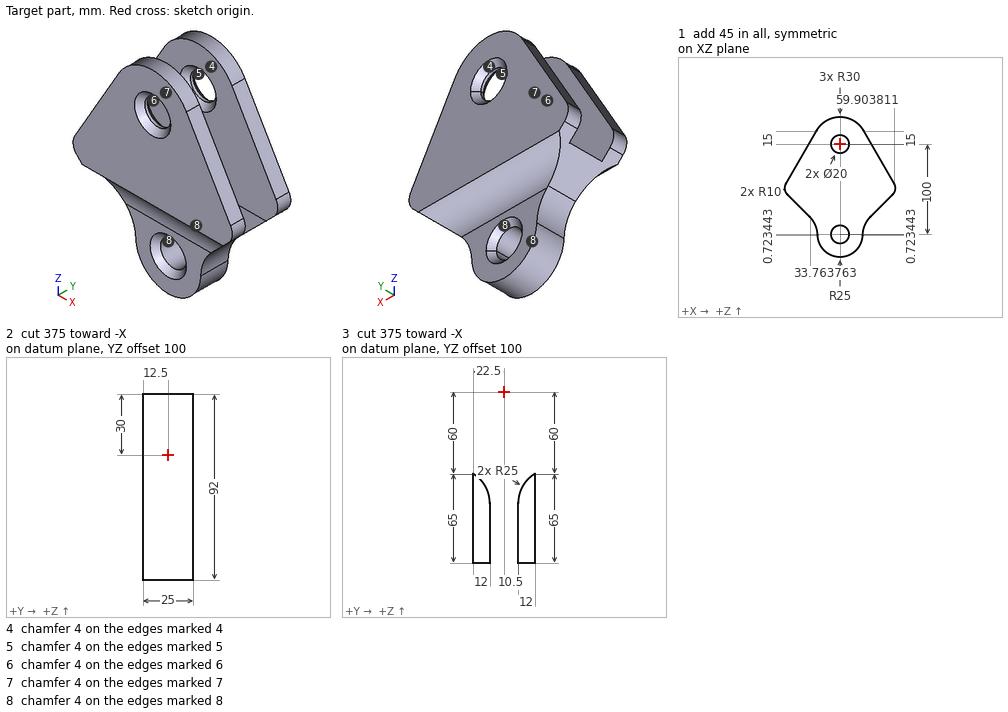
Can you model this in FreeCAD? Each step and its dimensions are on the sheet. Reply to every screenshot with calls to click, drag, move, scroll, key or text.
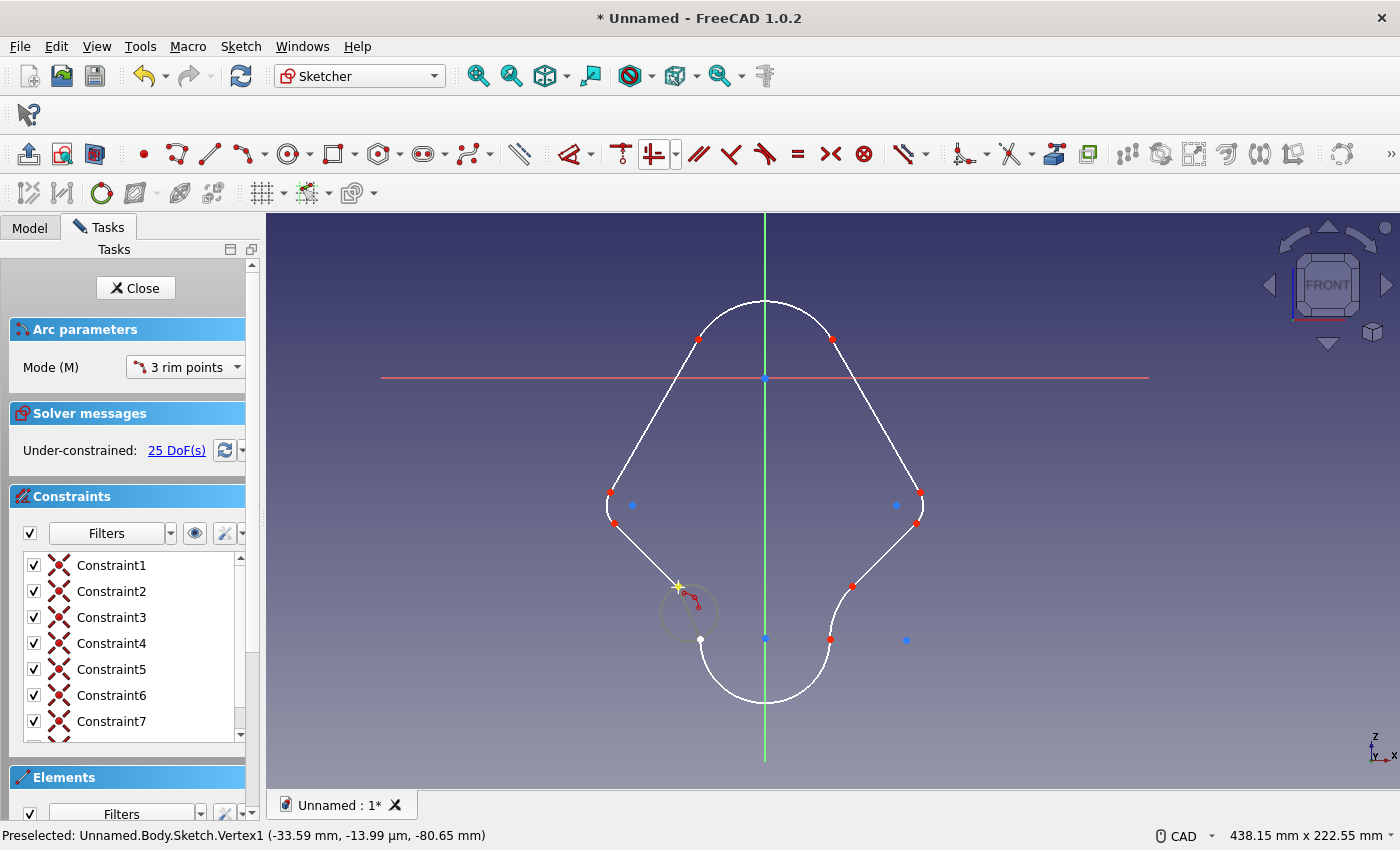
scroll(694, 610, up, 6)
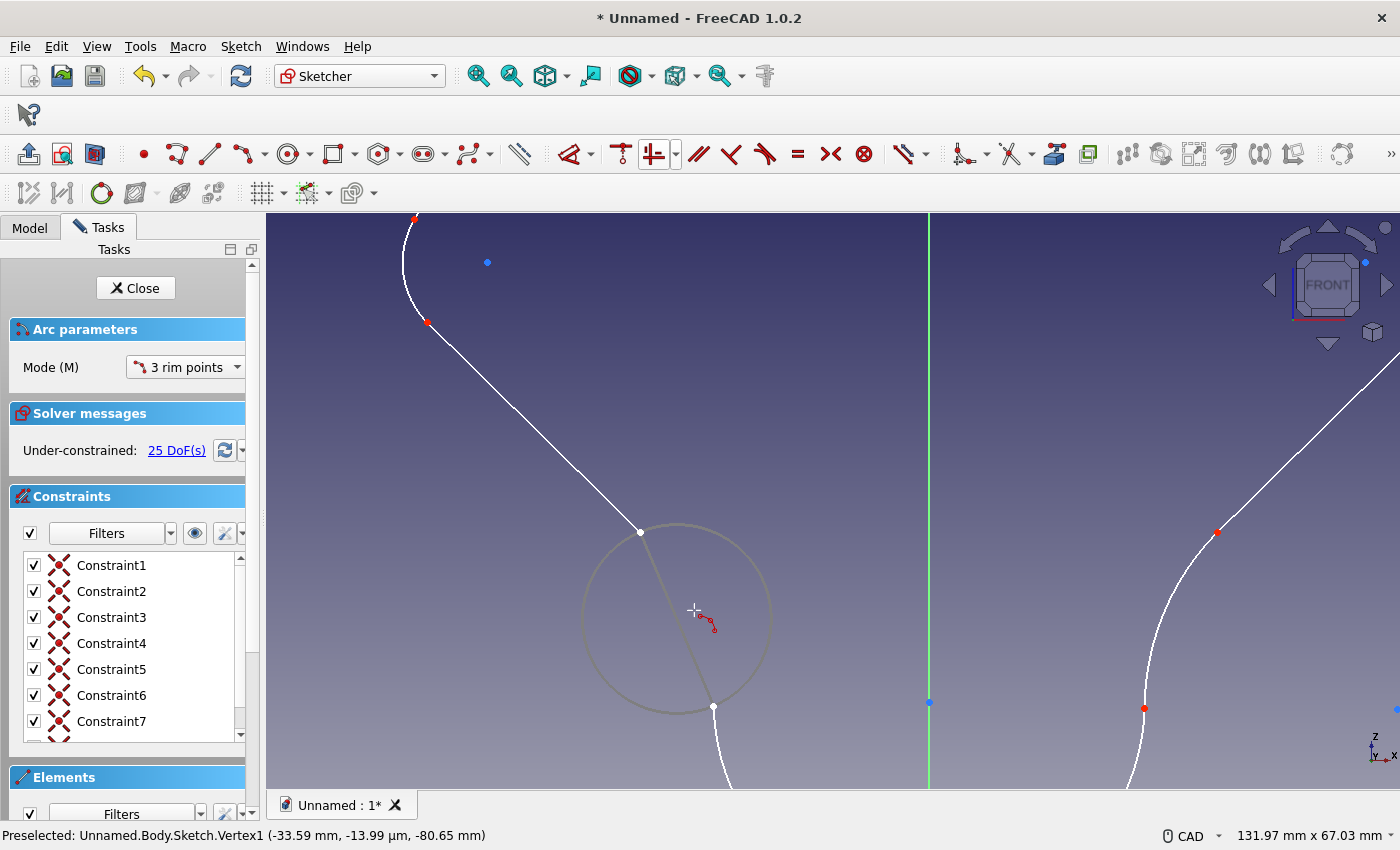
click(693, 610)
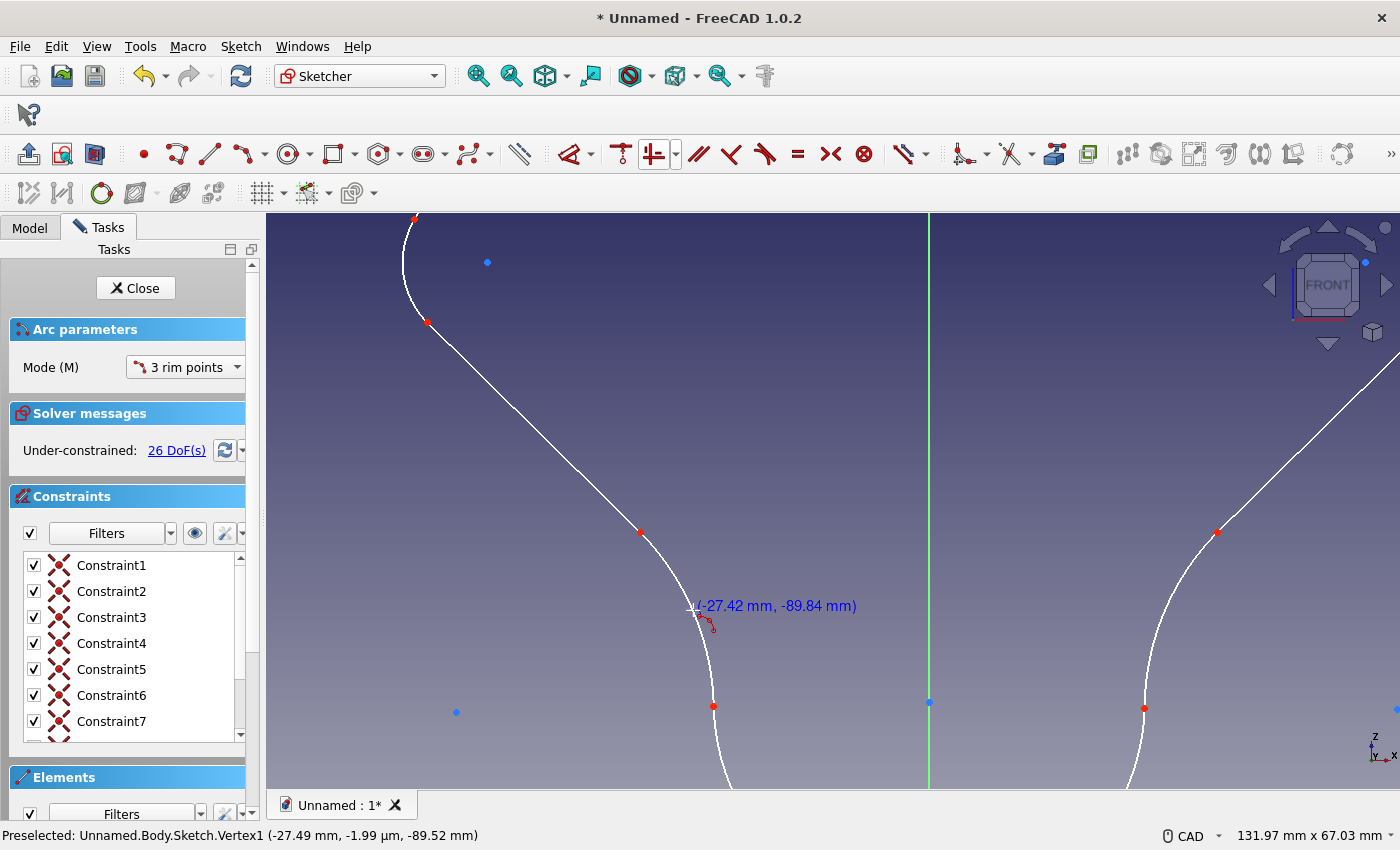
click(288, 154)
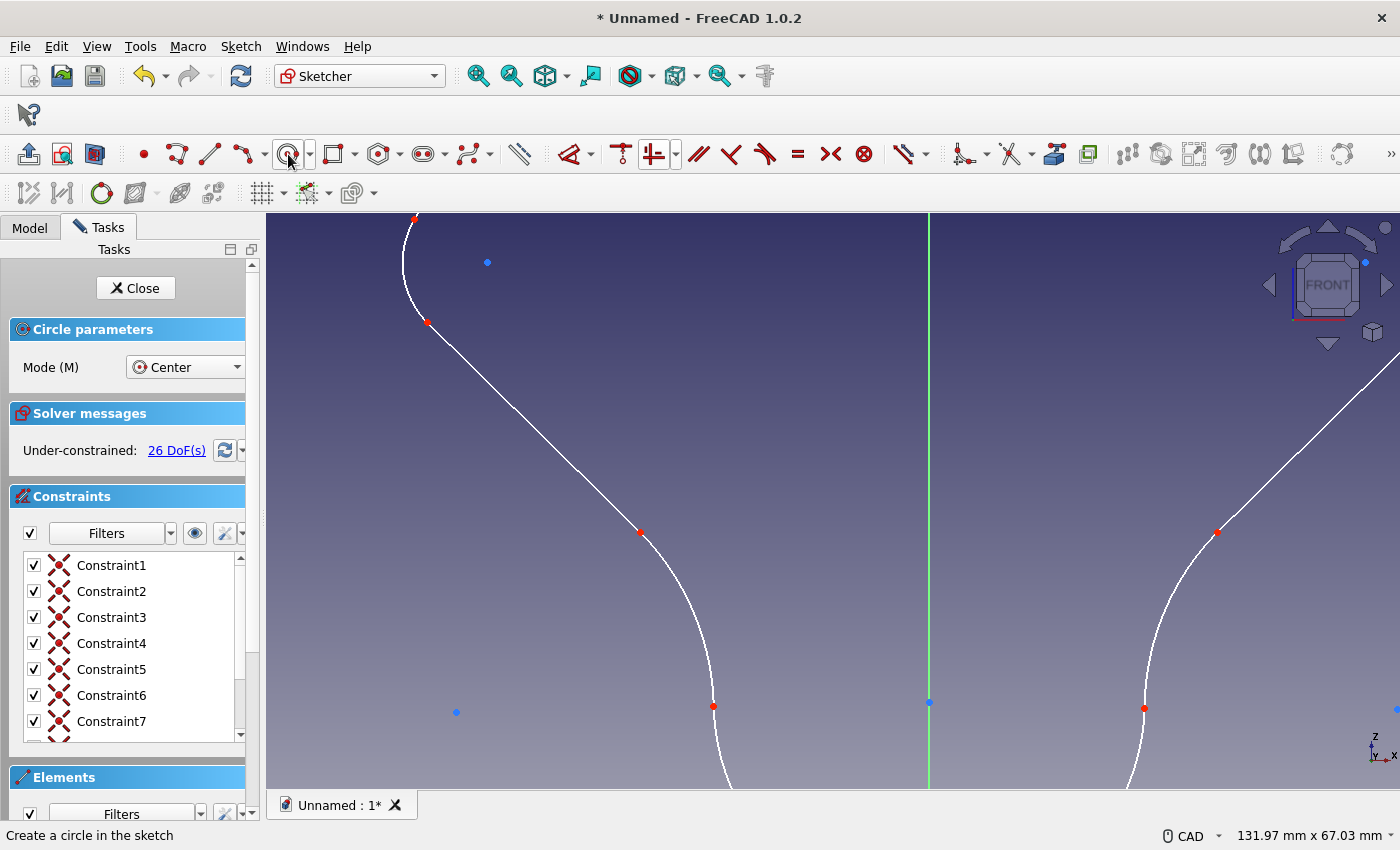
scroll(694, 610, down, 6)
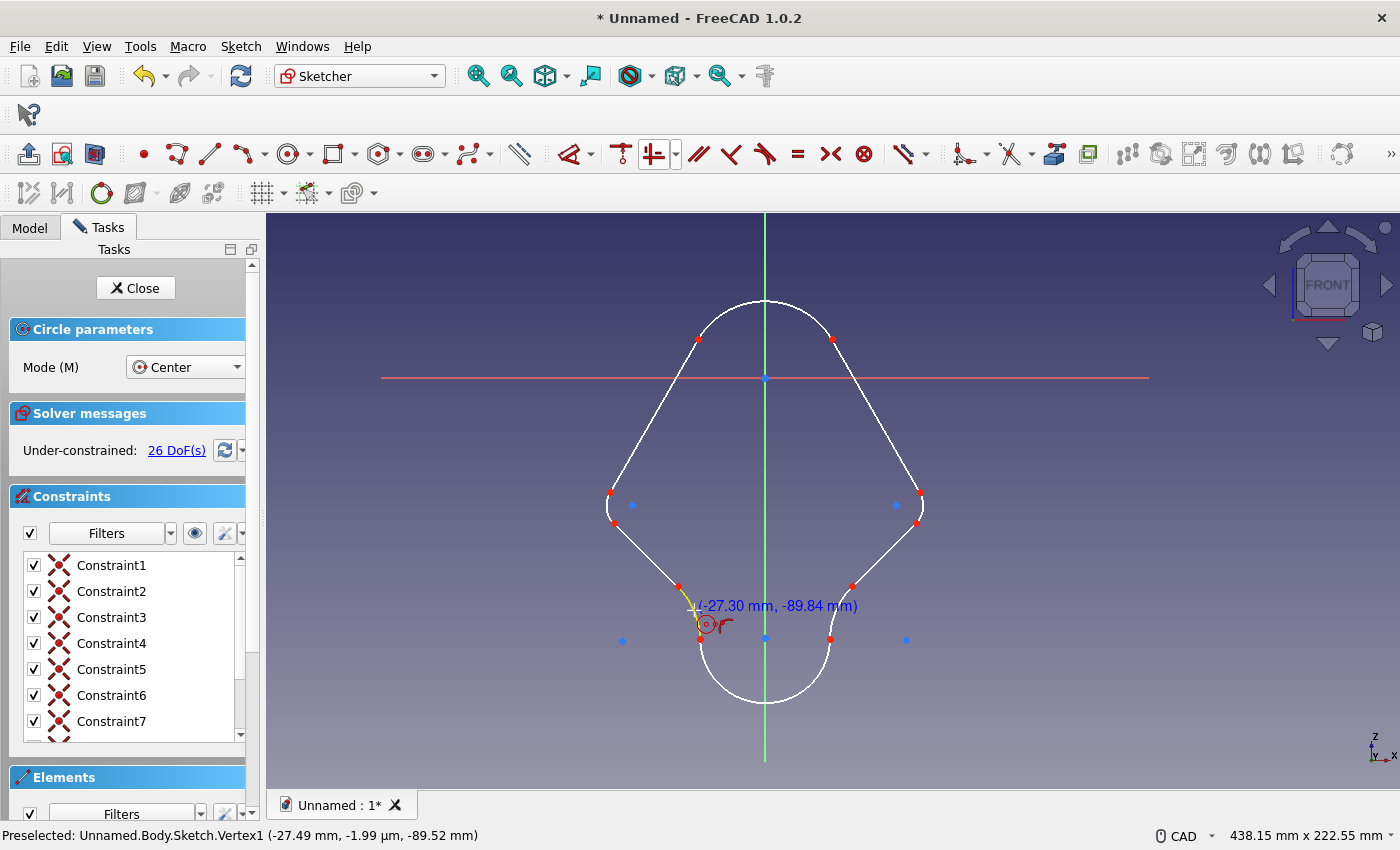
click(765, 378)
move(783, 360)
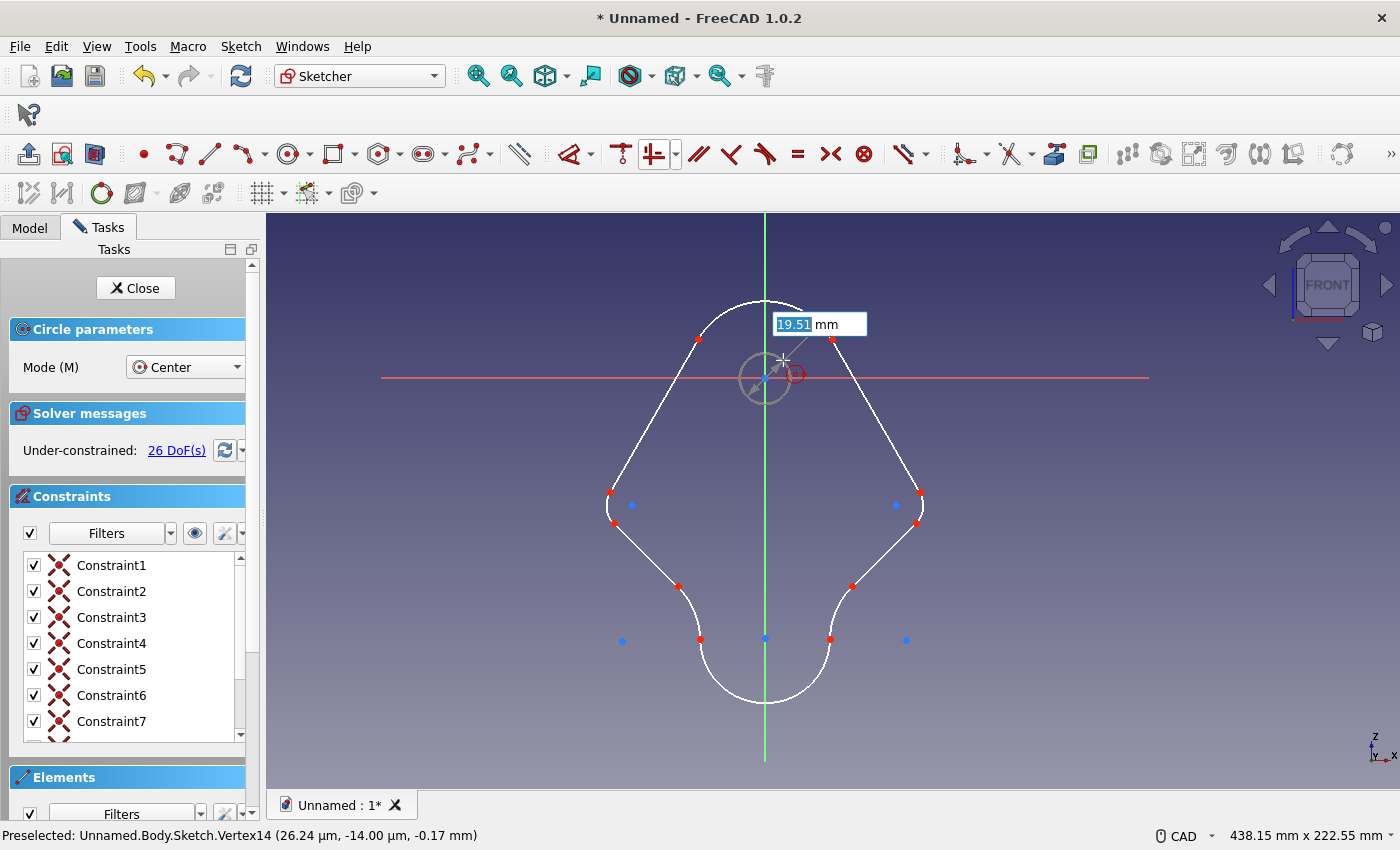
text(20)
key(Return)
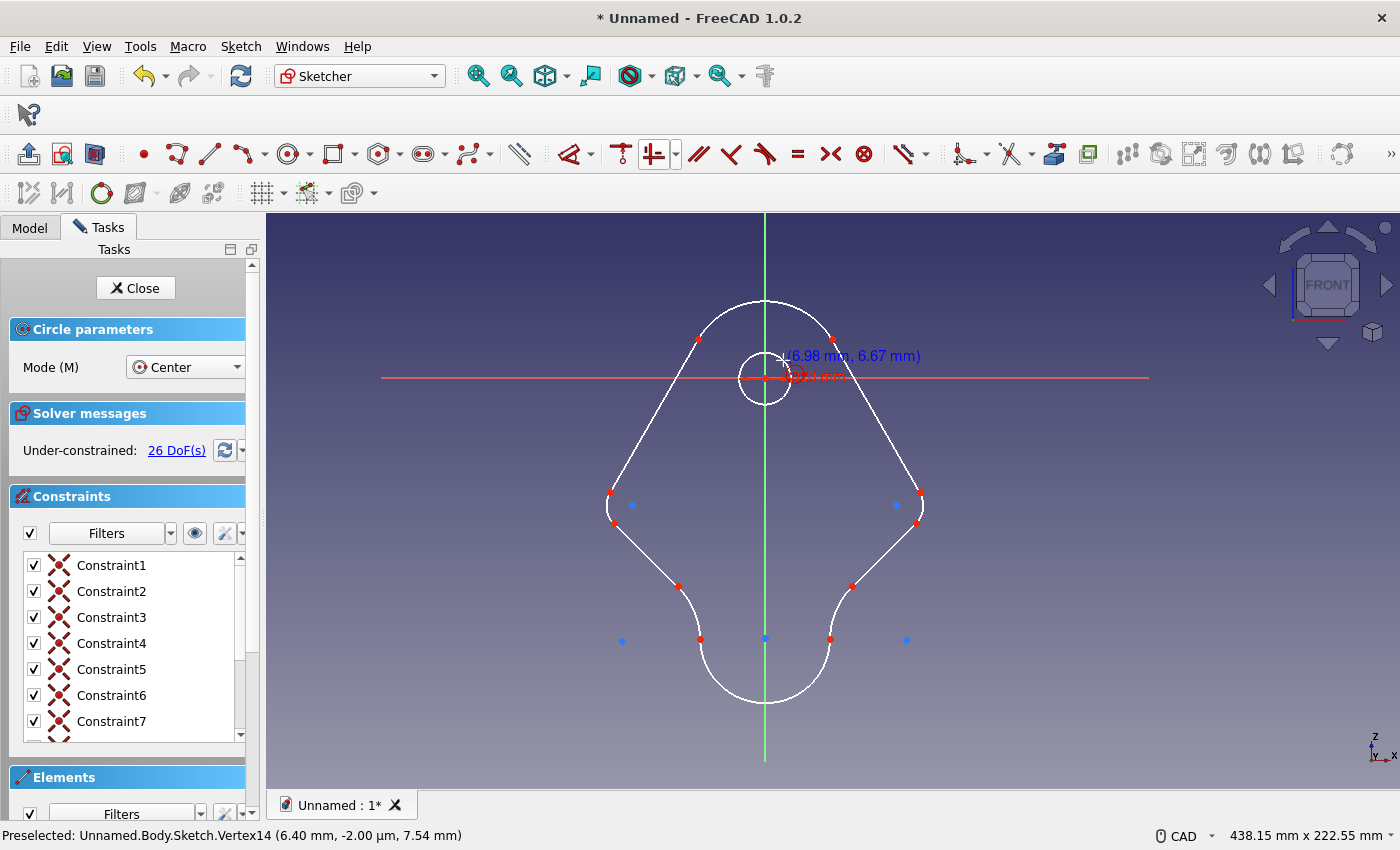
click(765, 637)
move(783, 619)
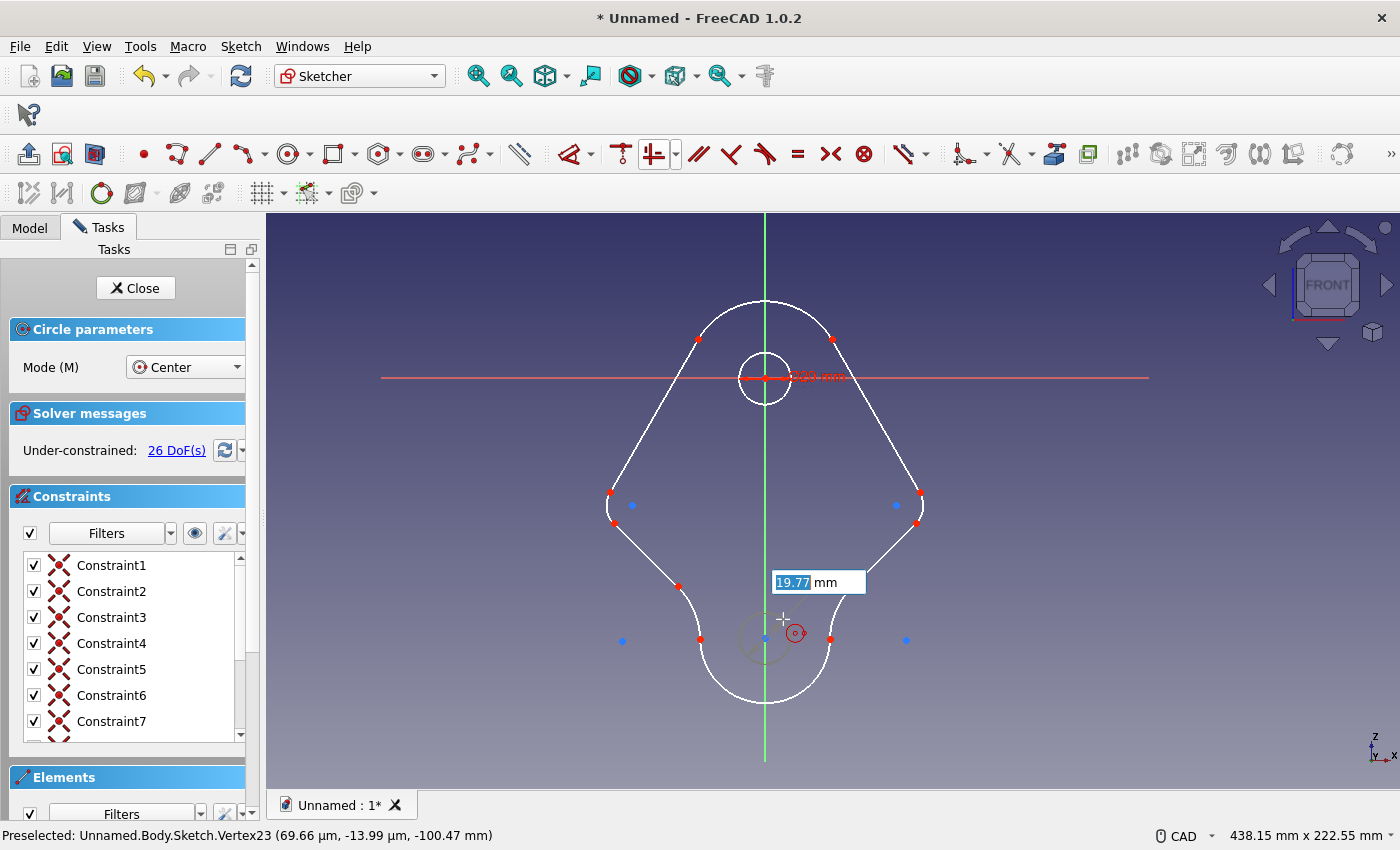
text(20)
key(Return)
key(Escape)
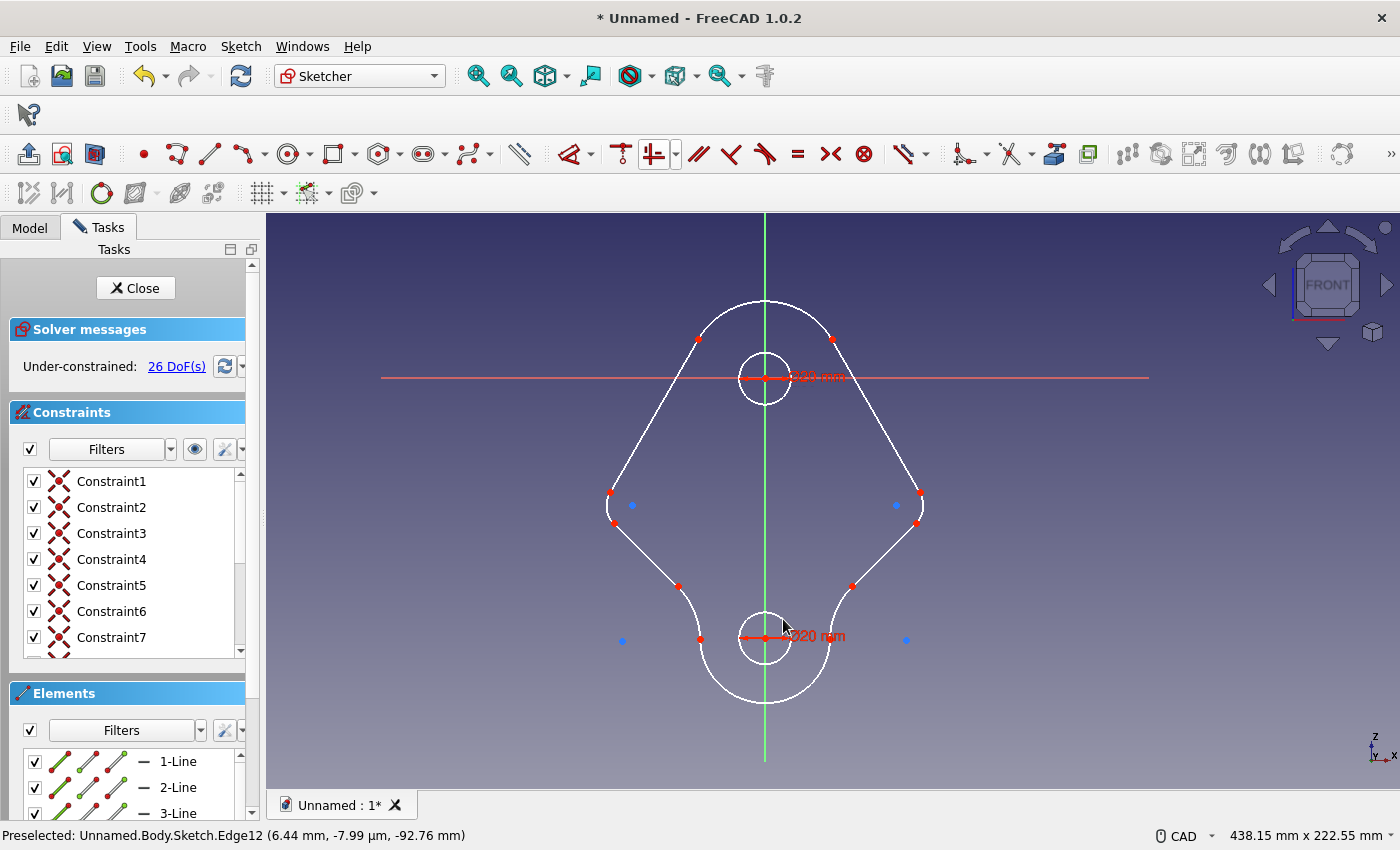
click(659, 568)